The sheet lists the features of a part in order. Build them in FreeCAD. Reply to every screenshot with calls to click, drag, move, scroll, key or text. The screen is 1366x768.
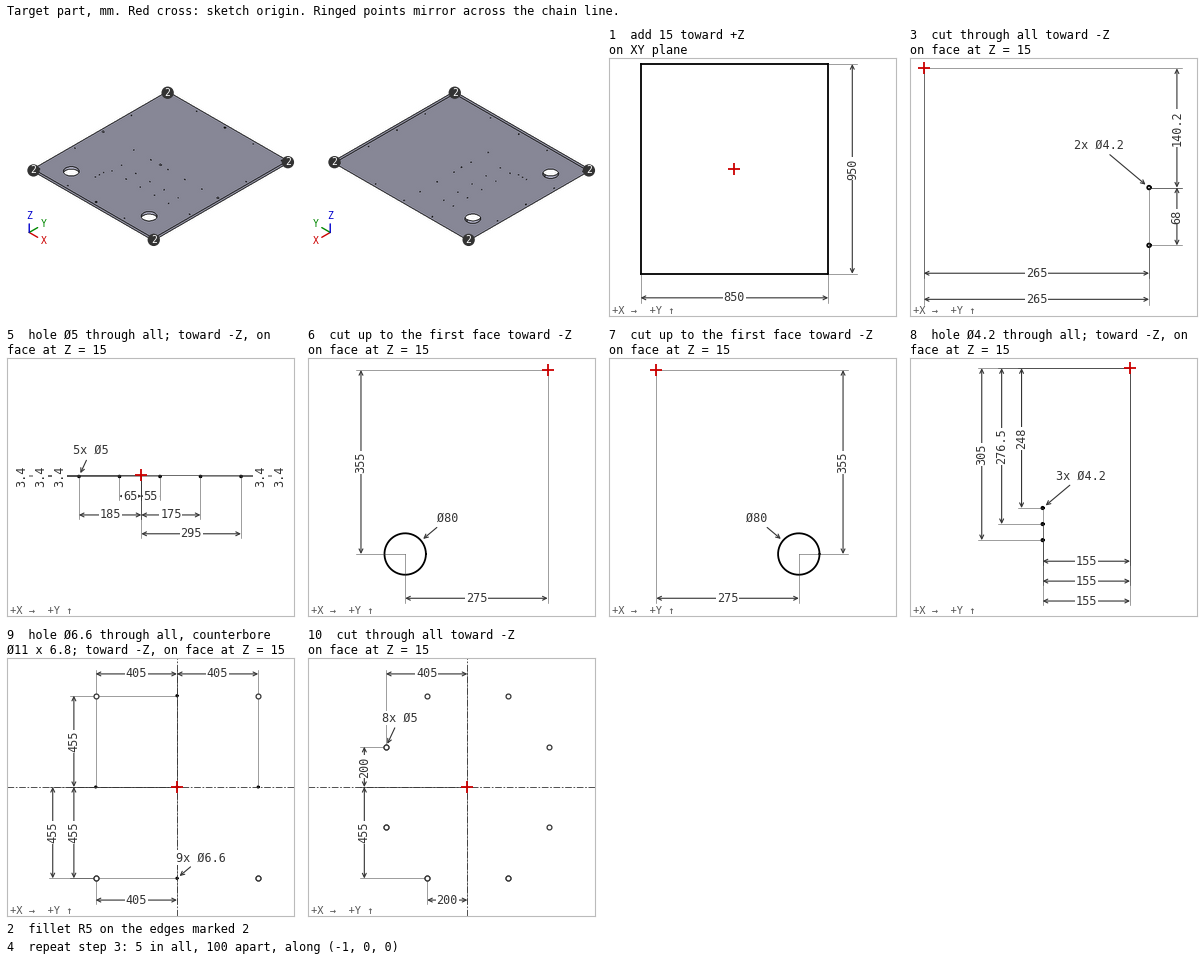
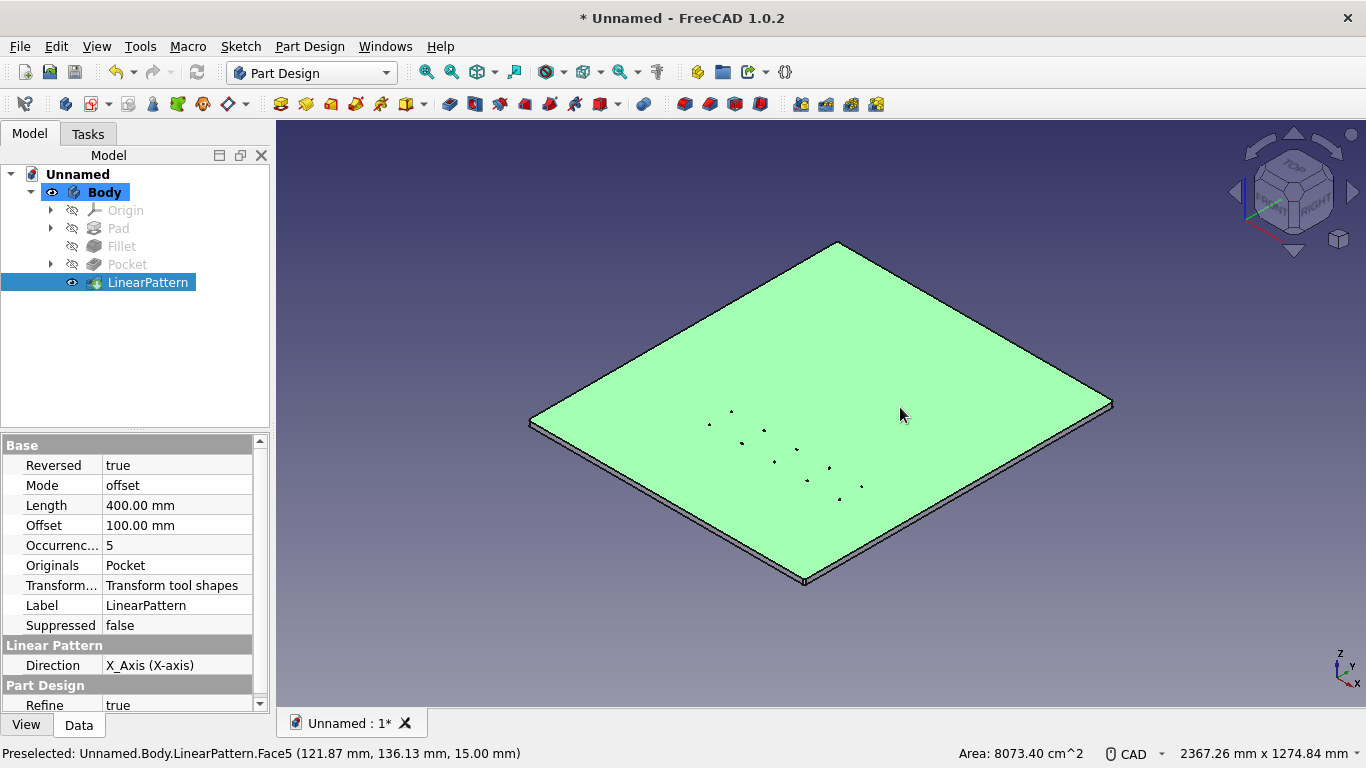
click(90, 104)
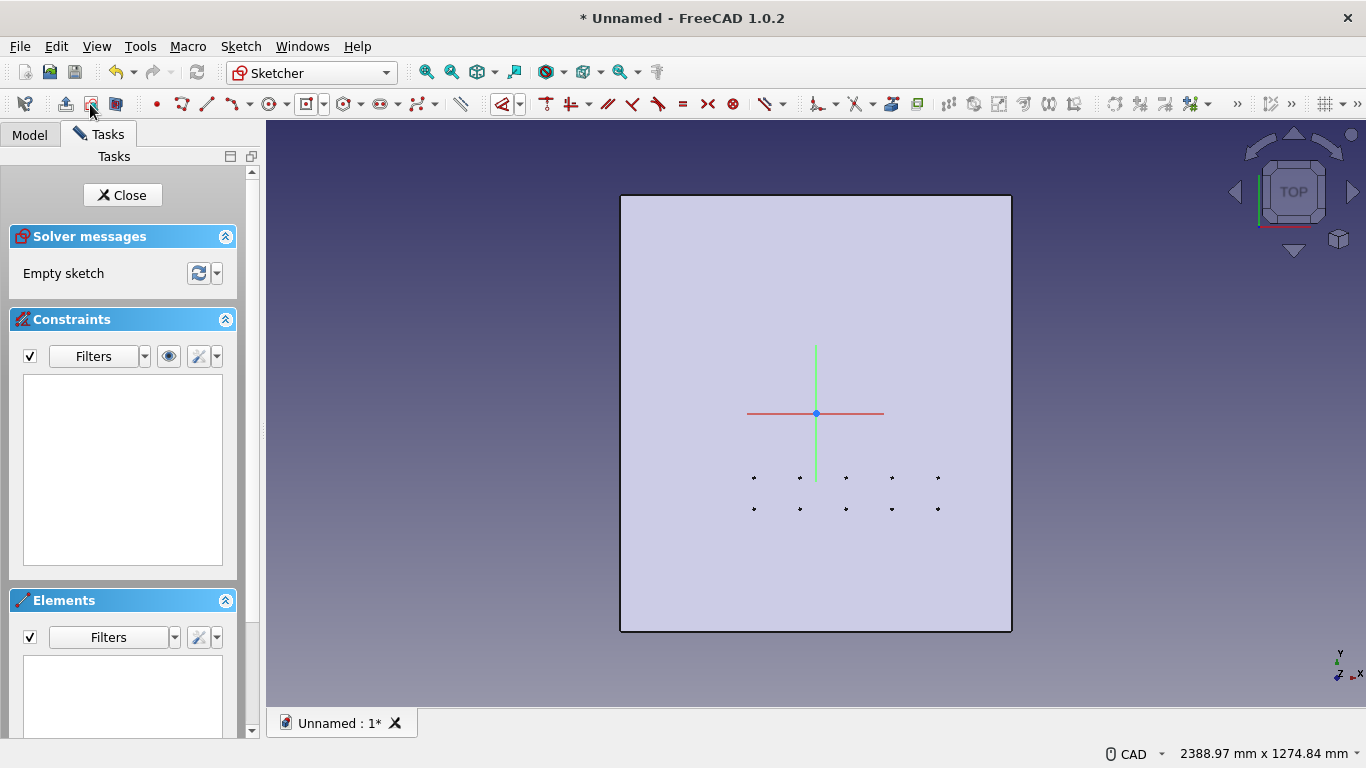
scroll(896, 416, up, 5)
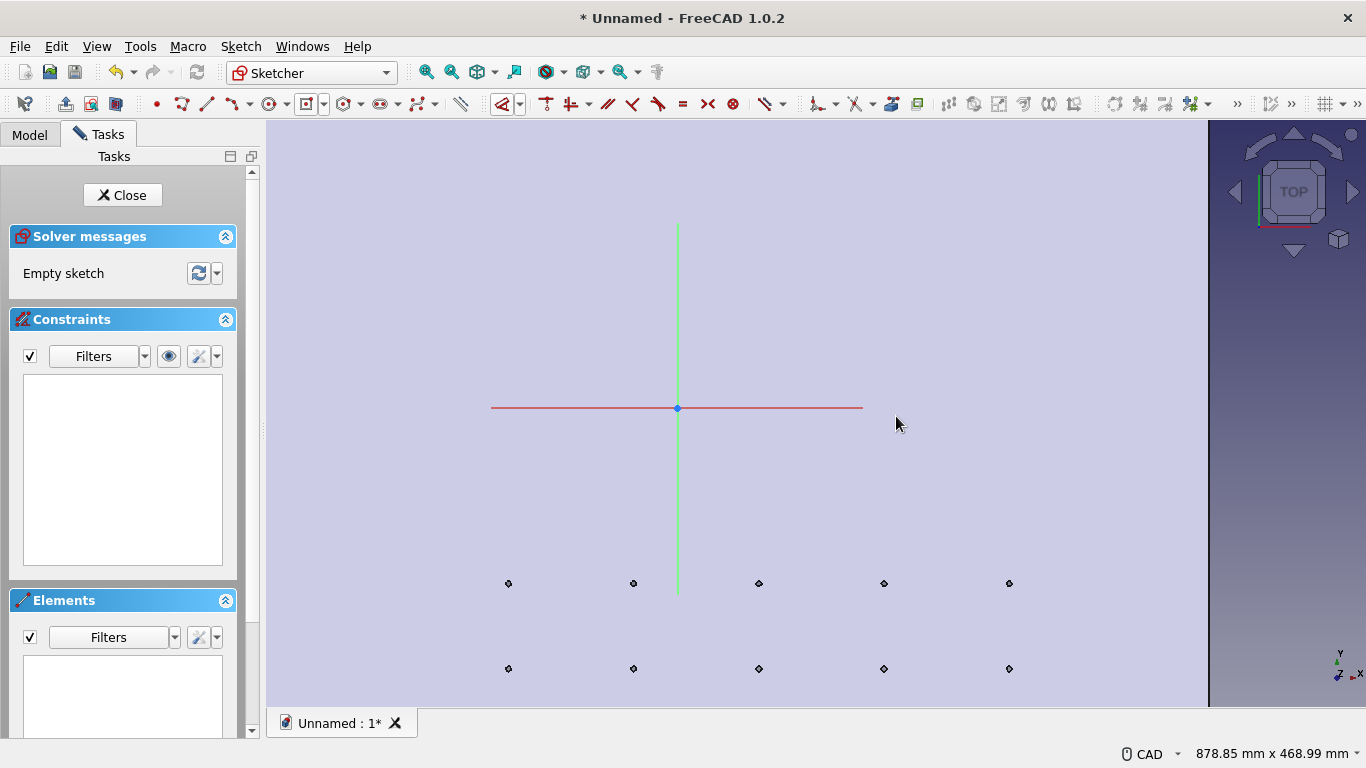
click(268, 104)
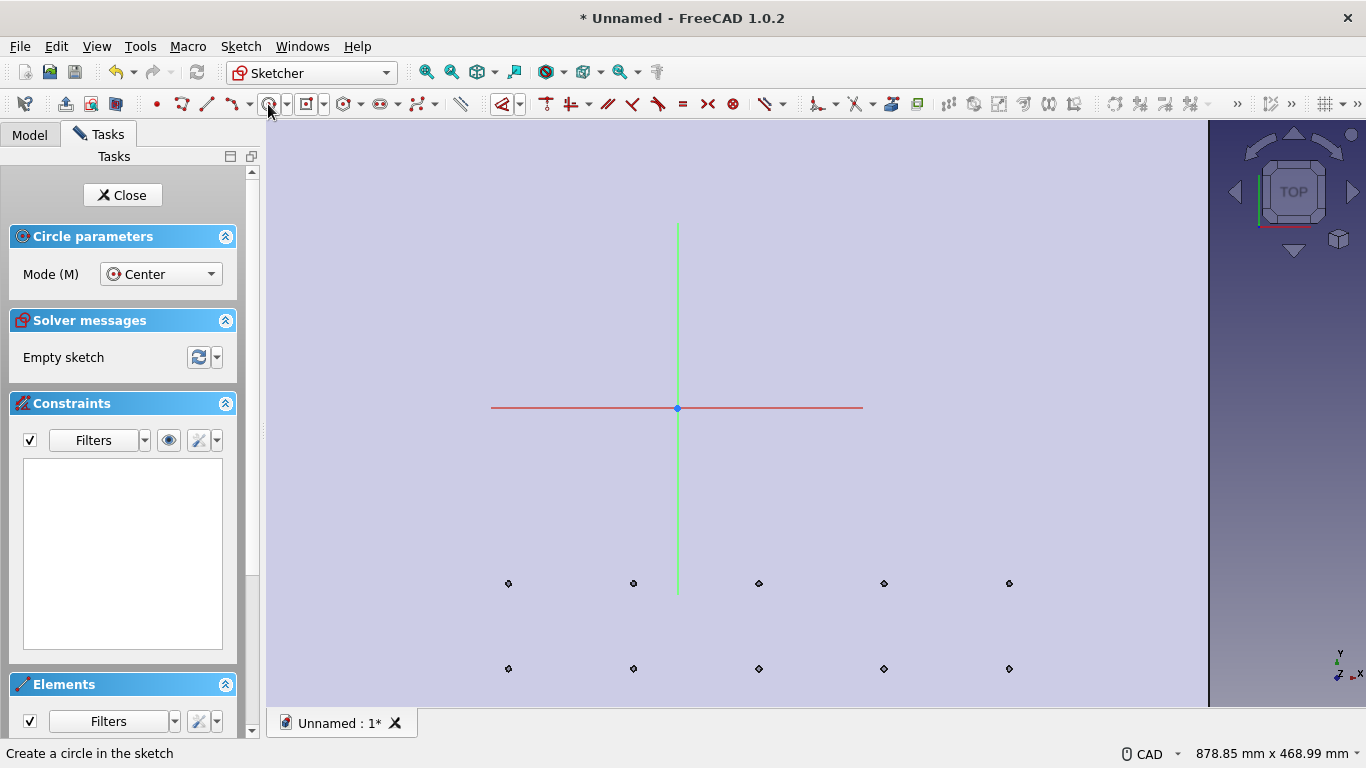
scroll(446, 413, up, 10)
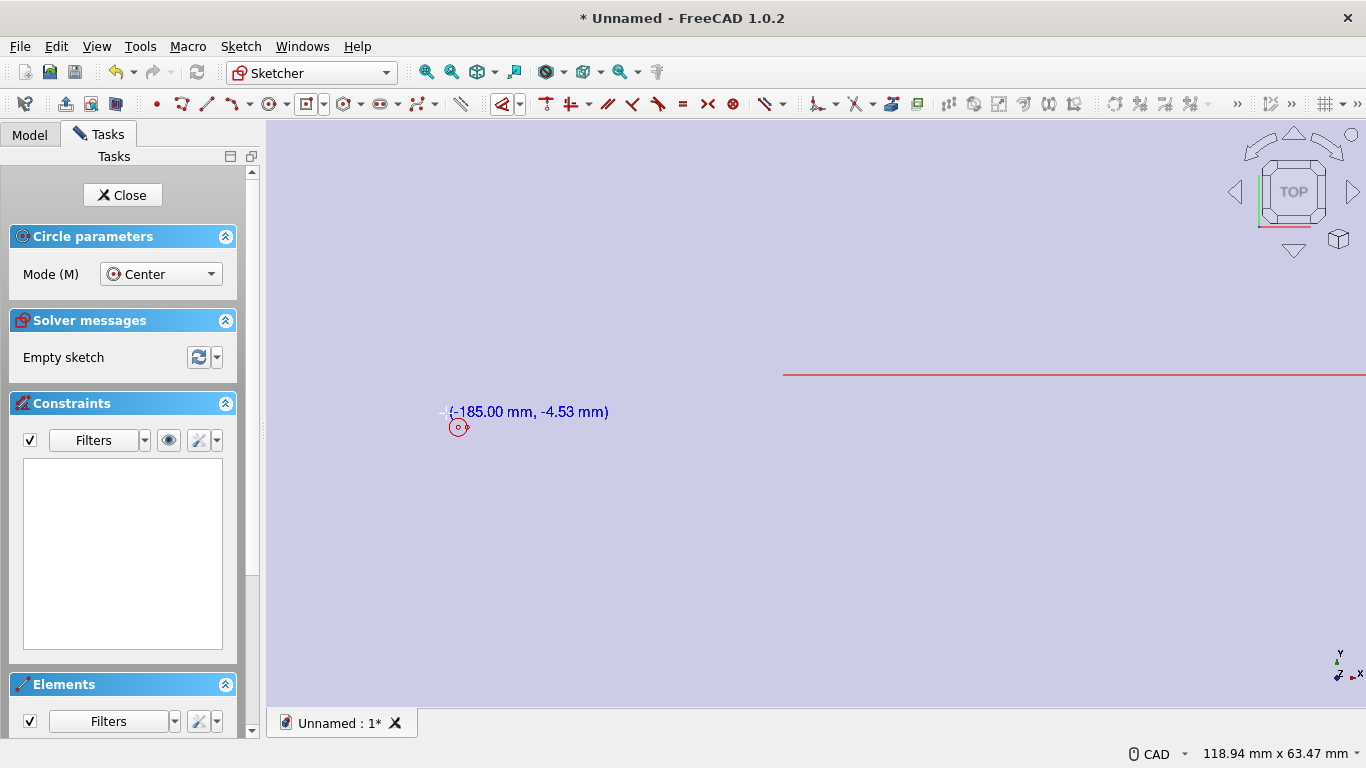
click(445, 407)
move(461, 390)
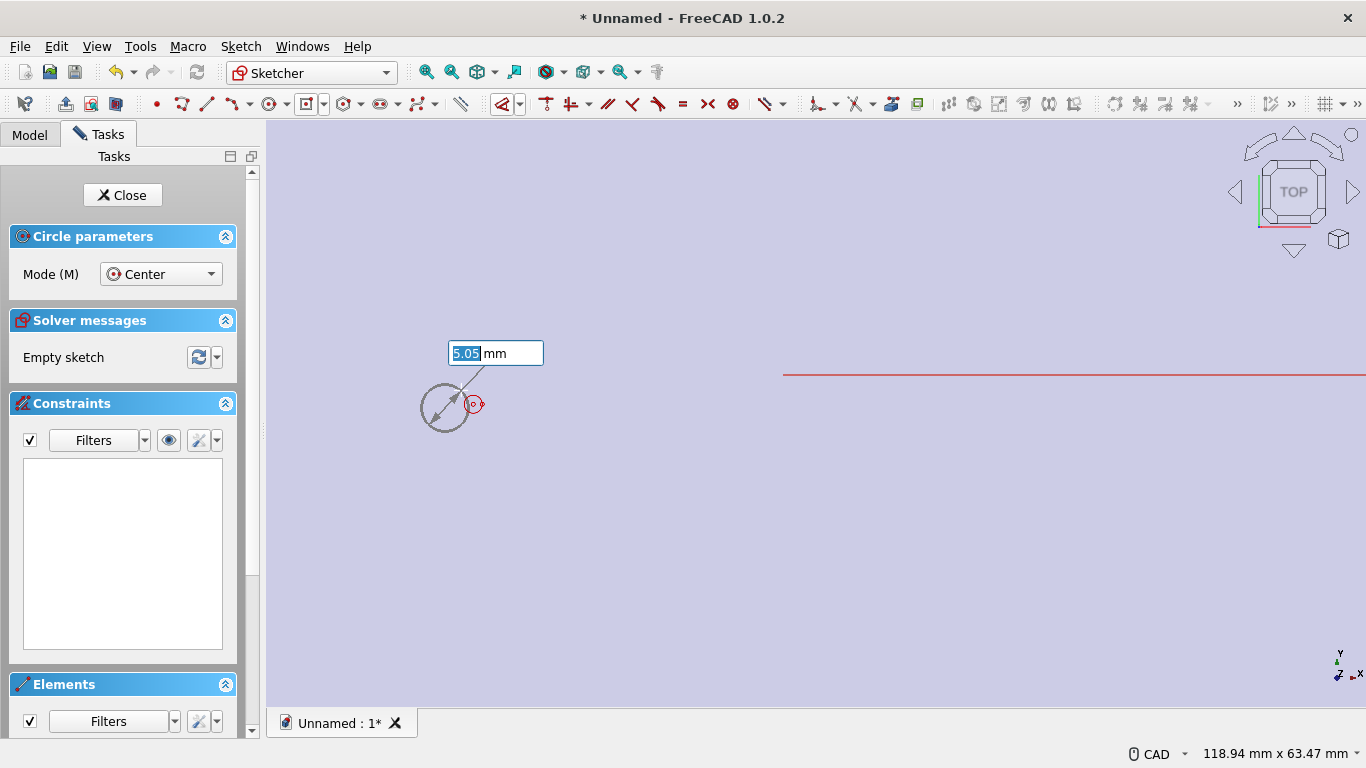
text(5)
key(Return)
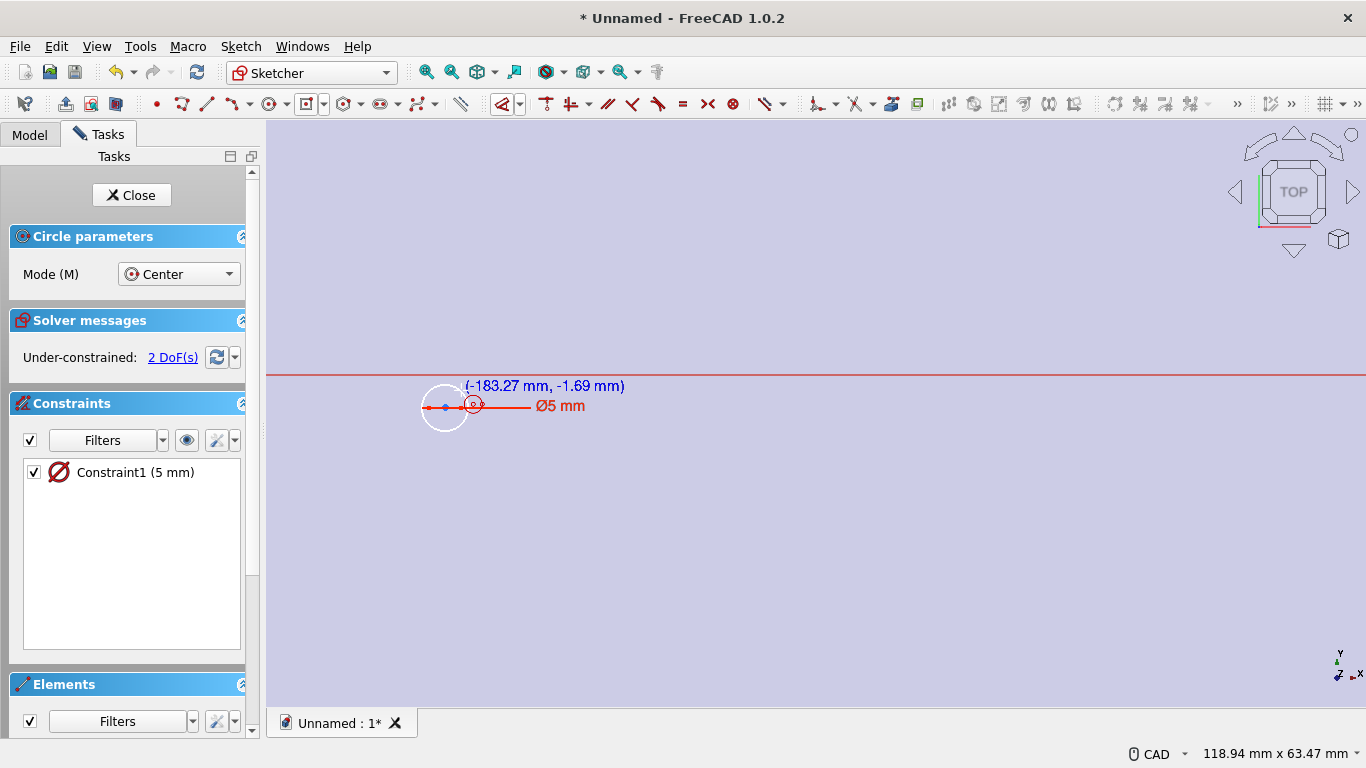
scroll(447, 415, down, 10)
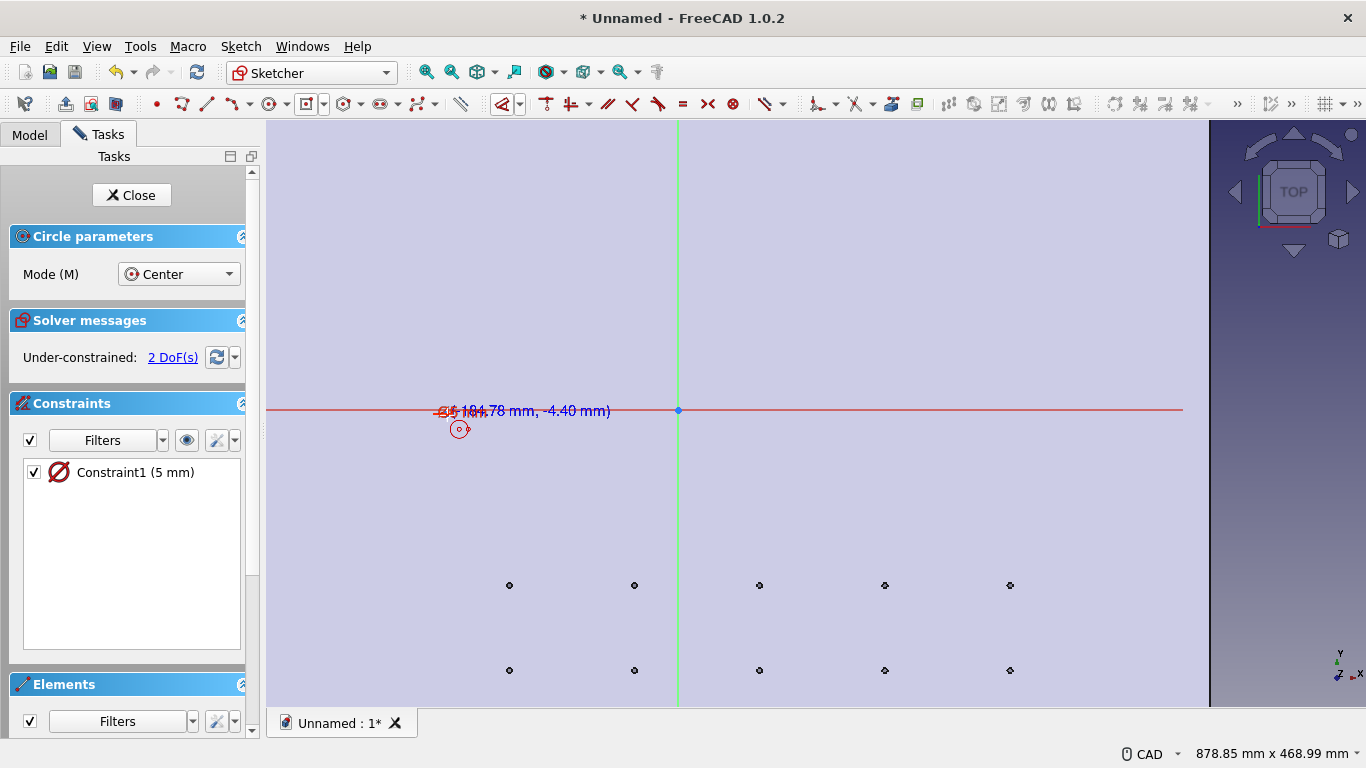
scroll(597, 414, up, 10)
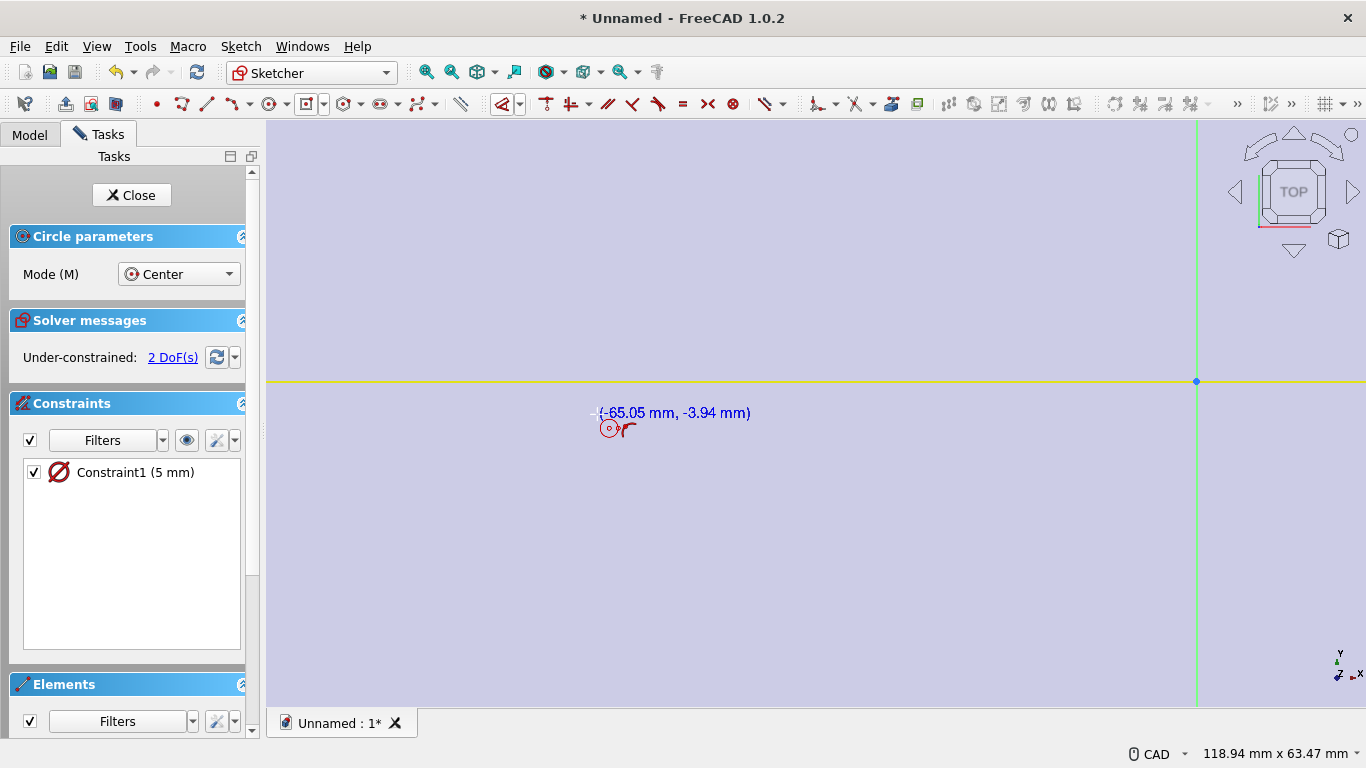
click(596, 413)
move(612, 397)